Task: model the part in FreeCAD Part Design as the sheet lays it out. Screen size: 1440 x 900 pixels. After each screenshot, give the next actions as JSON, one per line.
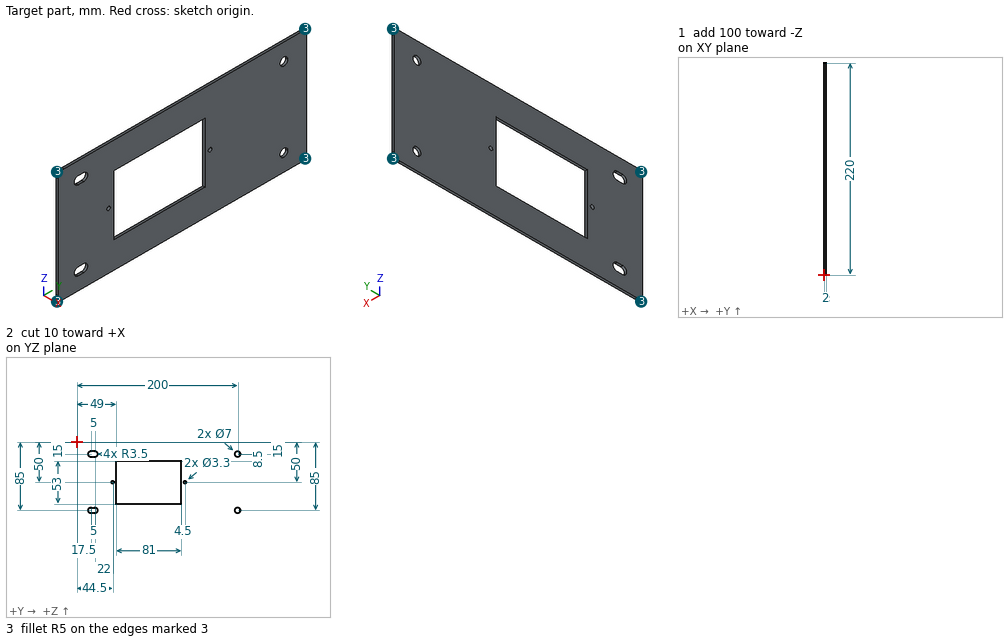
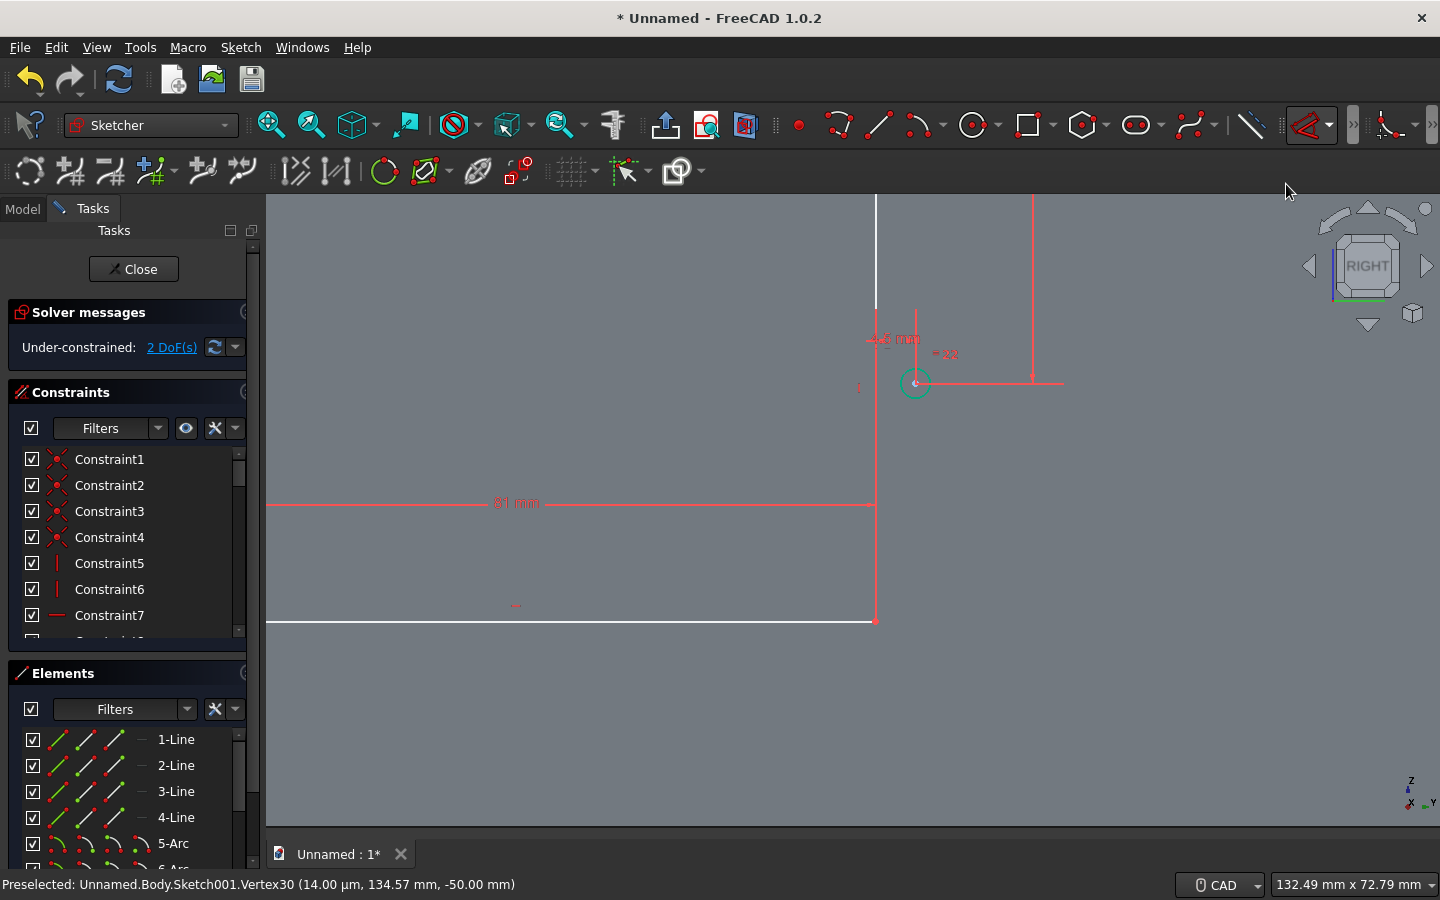
{"action": "scroll", "coordinate": [877, 624], "scroll_direction": "down", "scroll_amount": 5}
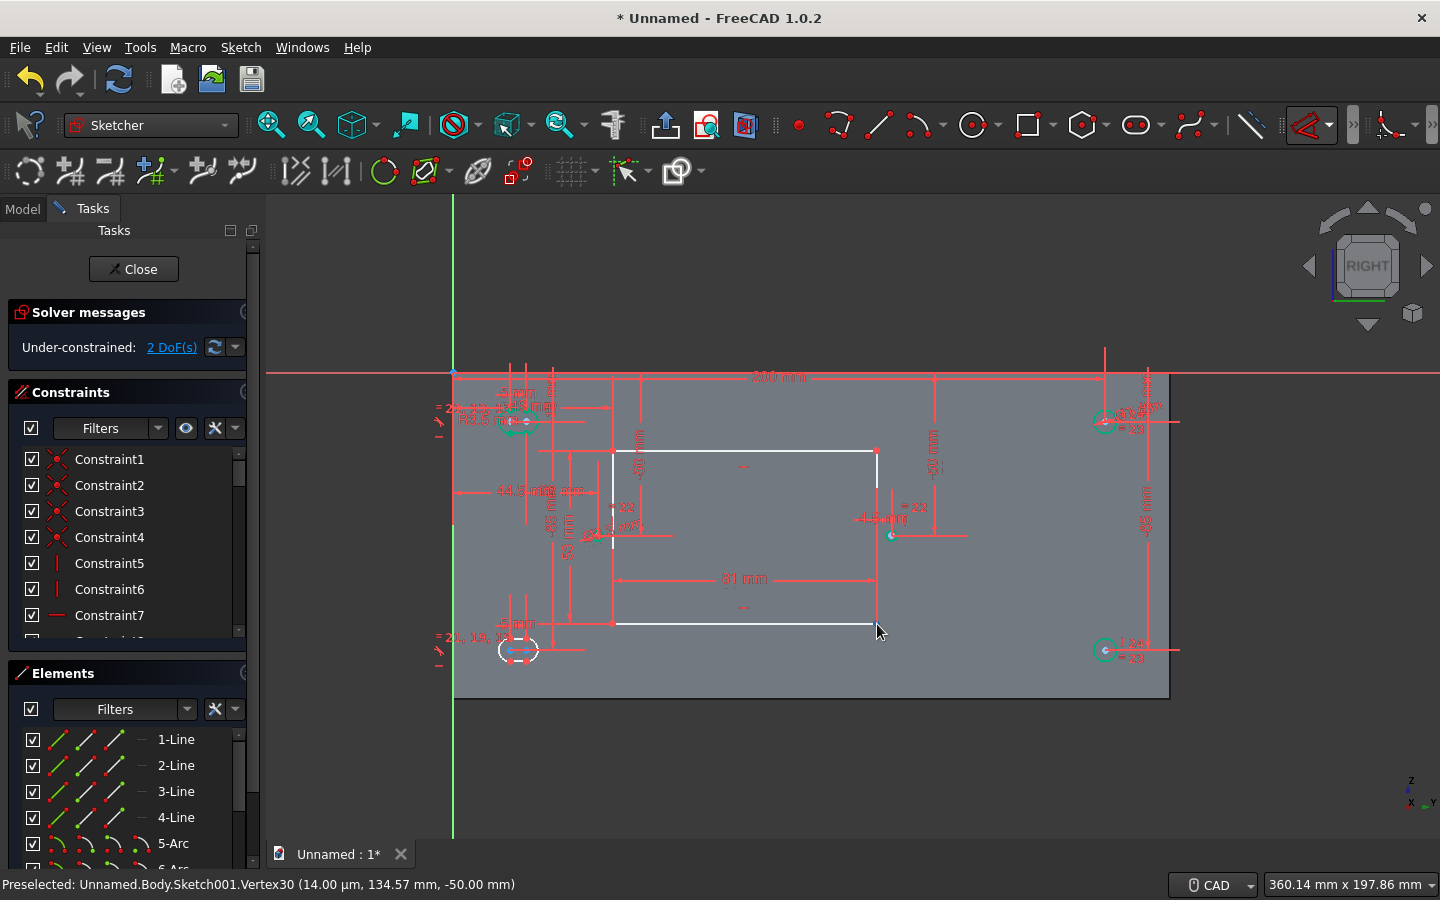
{"action": "scroll", "coordinate": [877, 451], "scroll_direction": "up", "scroll_amount": 2}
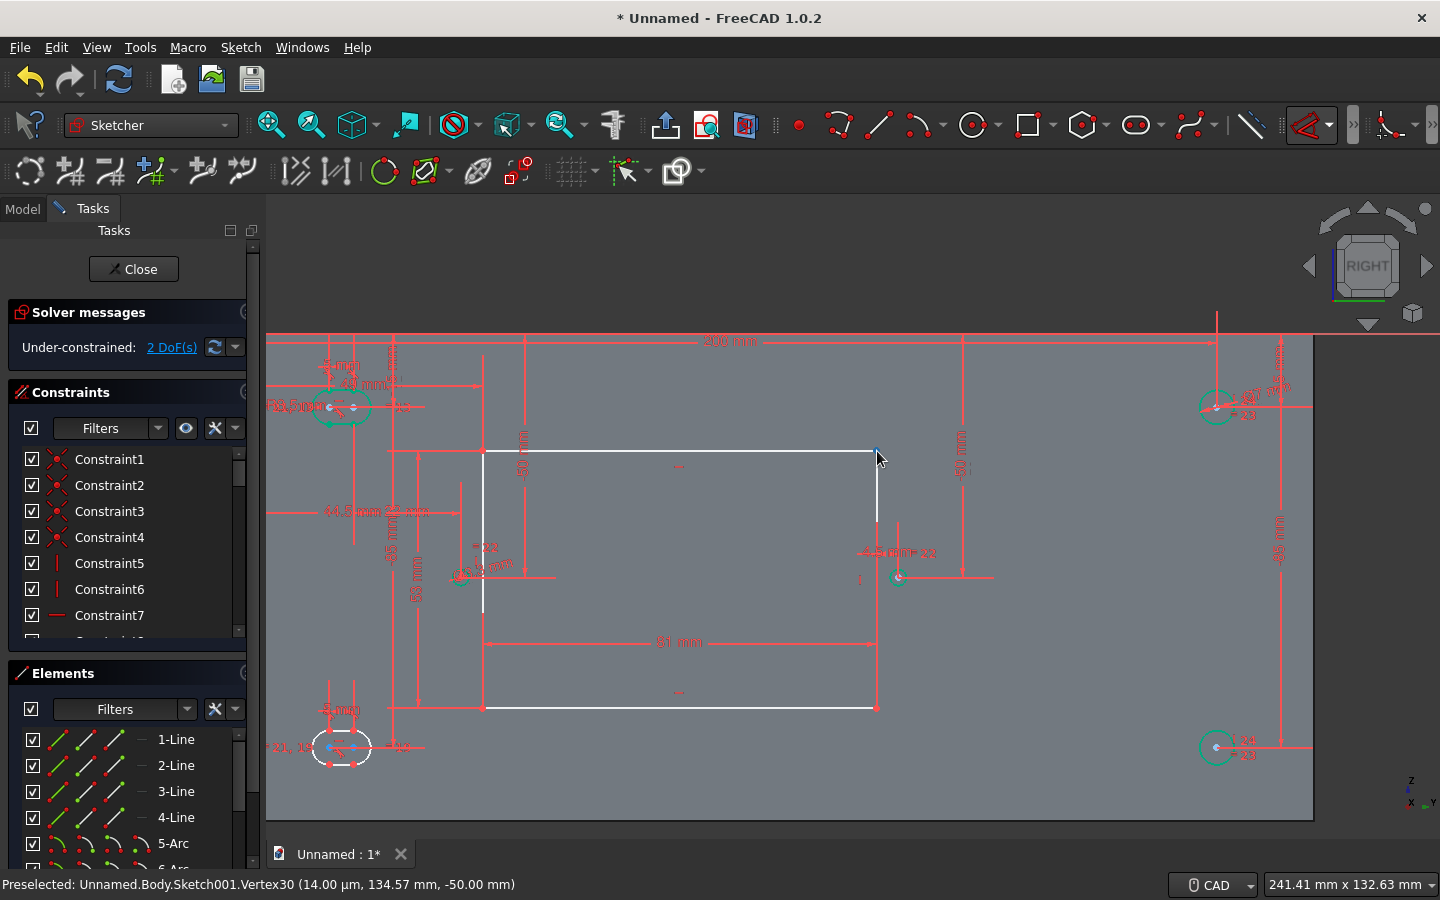
{"action": "left_click", "coordinate": [877, 451]}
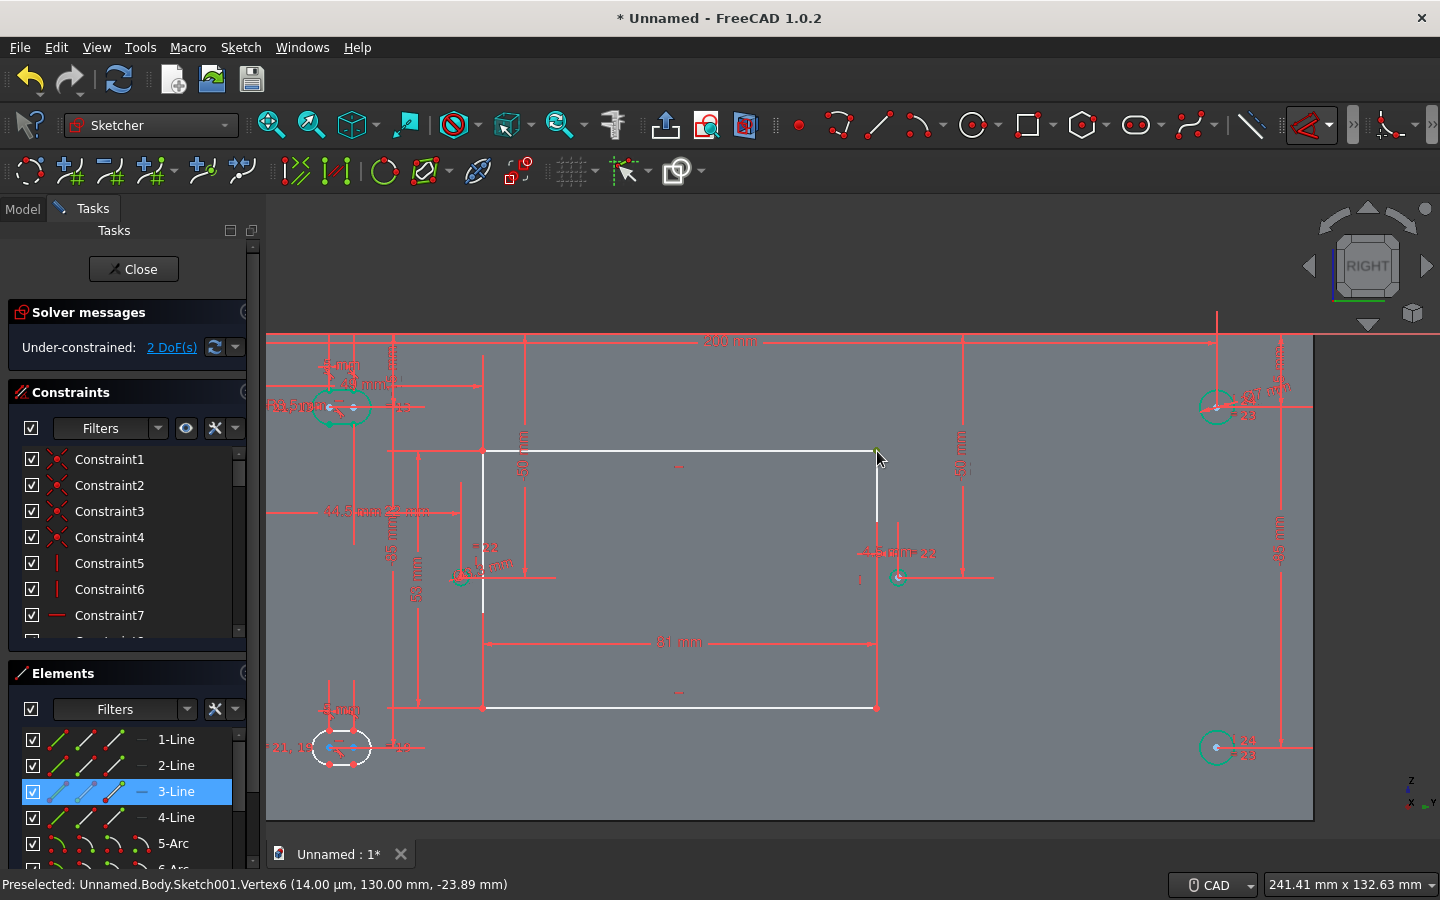
{"action": "left_click", "coordinate": [1217, 407]}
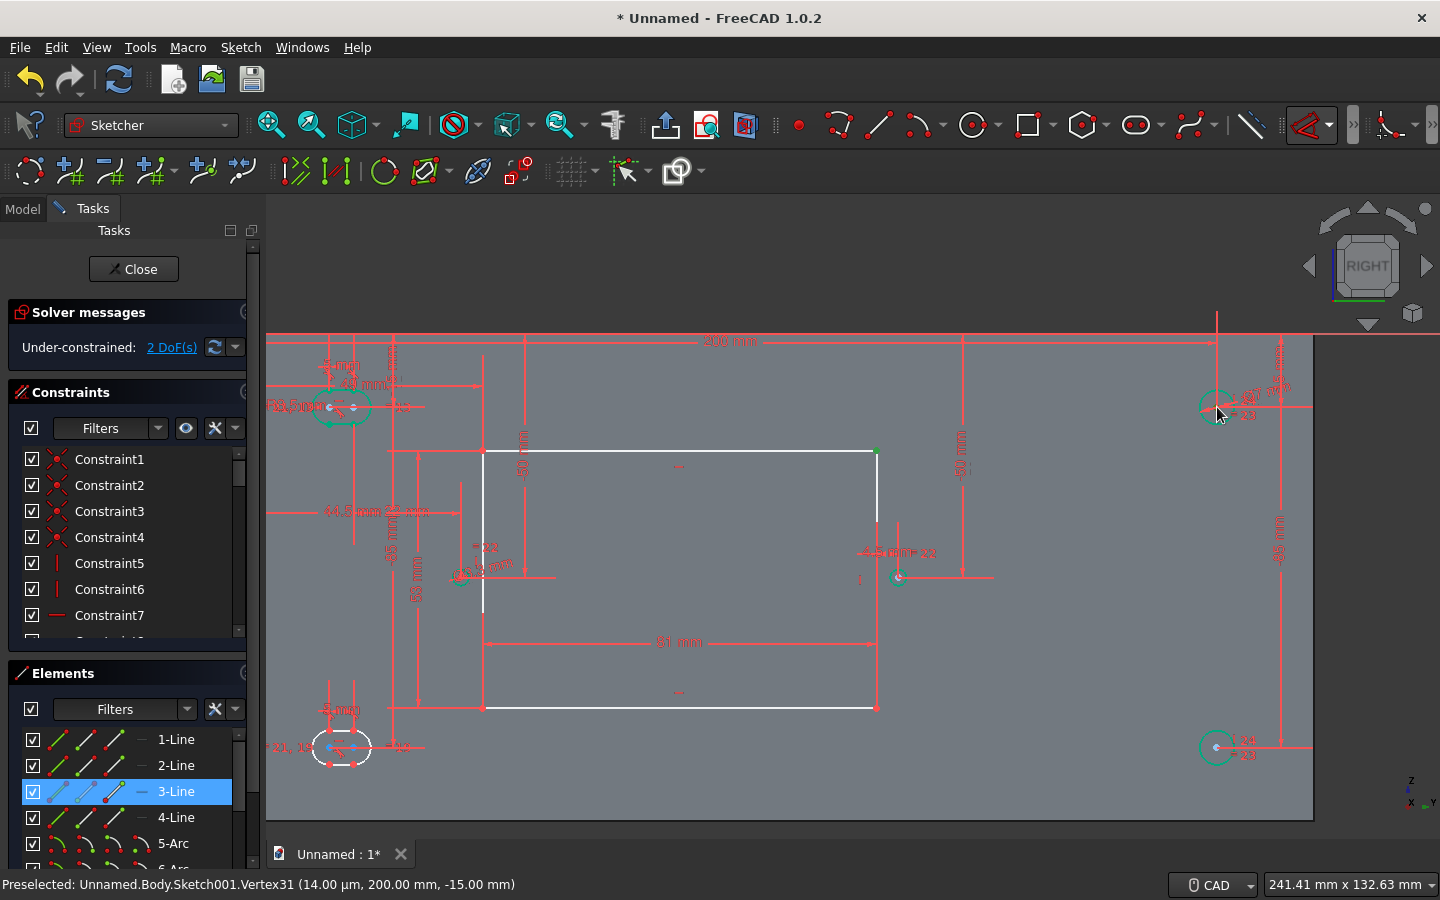
{"action": "key", "text": "i"}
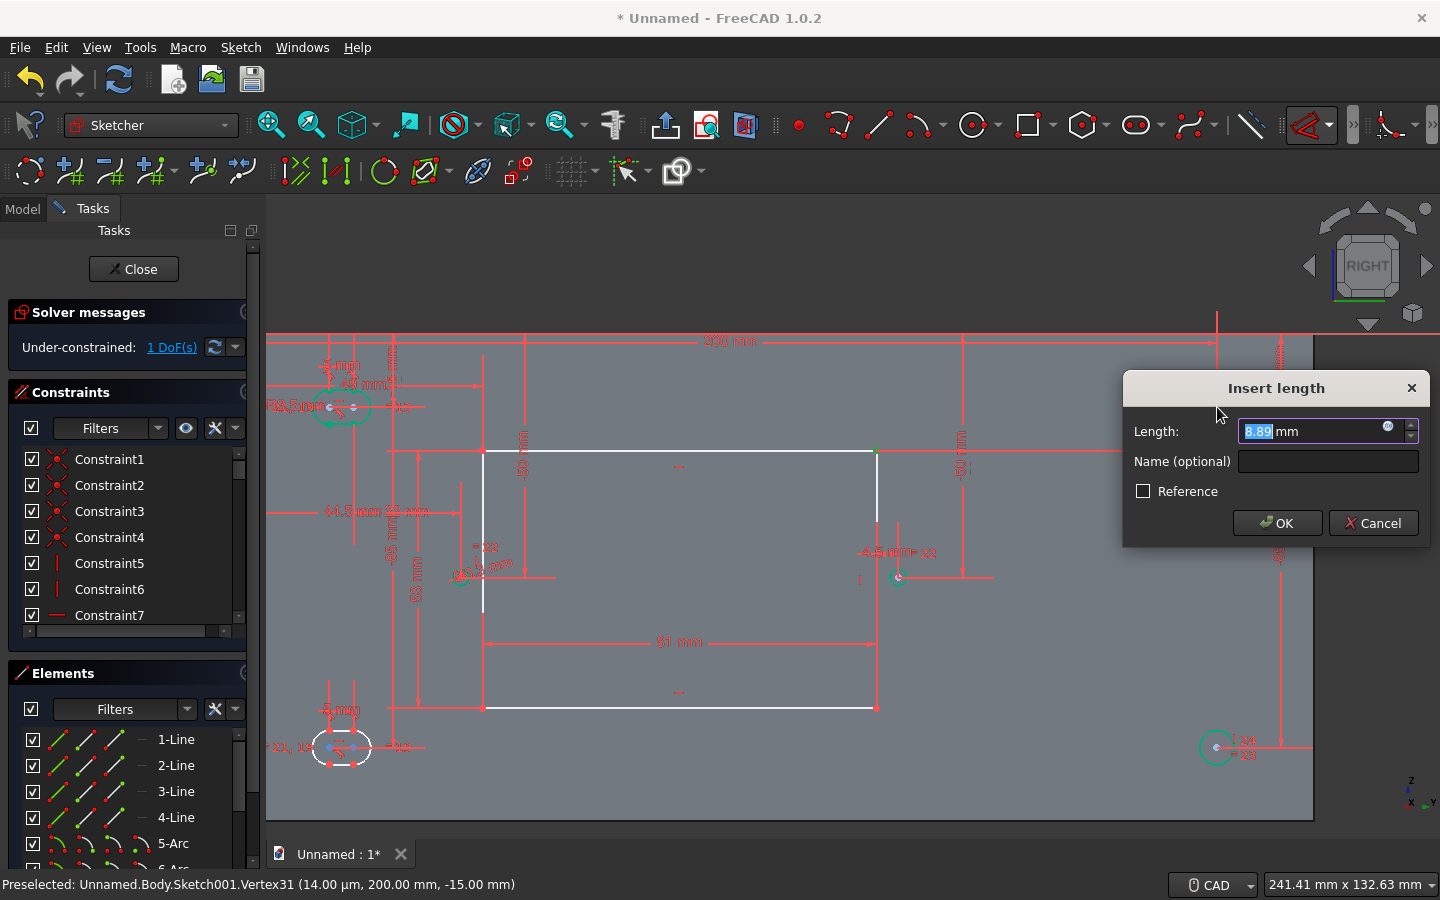
{"action": "type", "text": "8.5"}
{"action": "key", "text": "Return"}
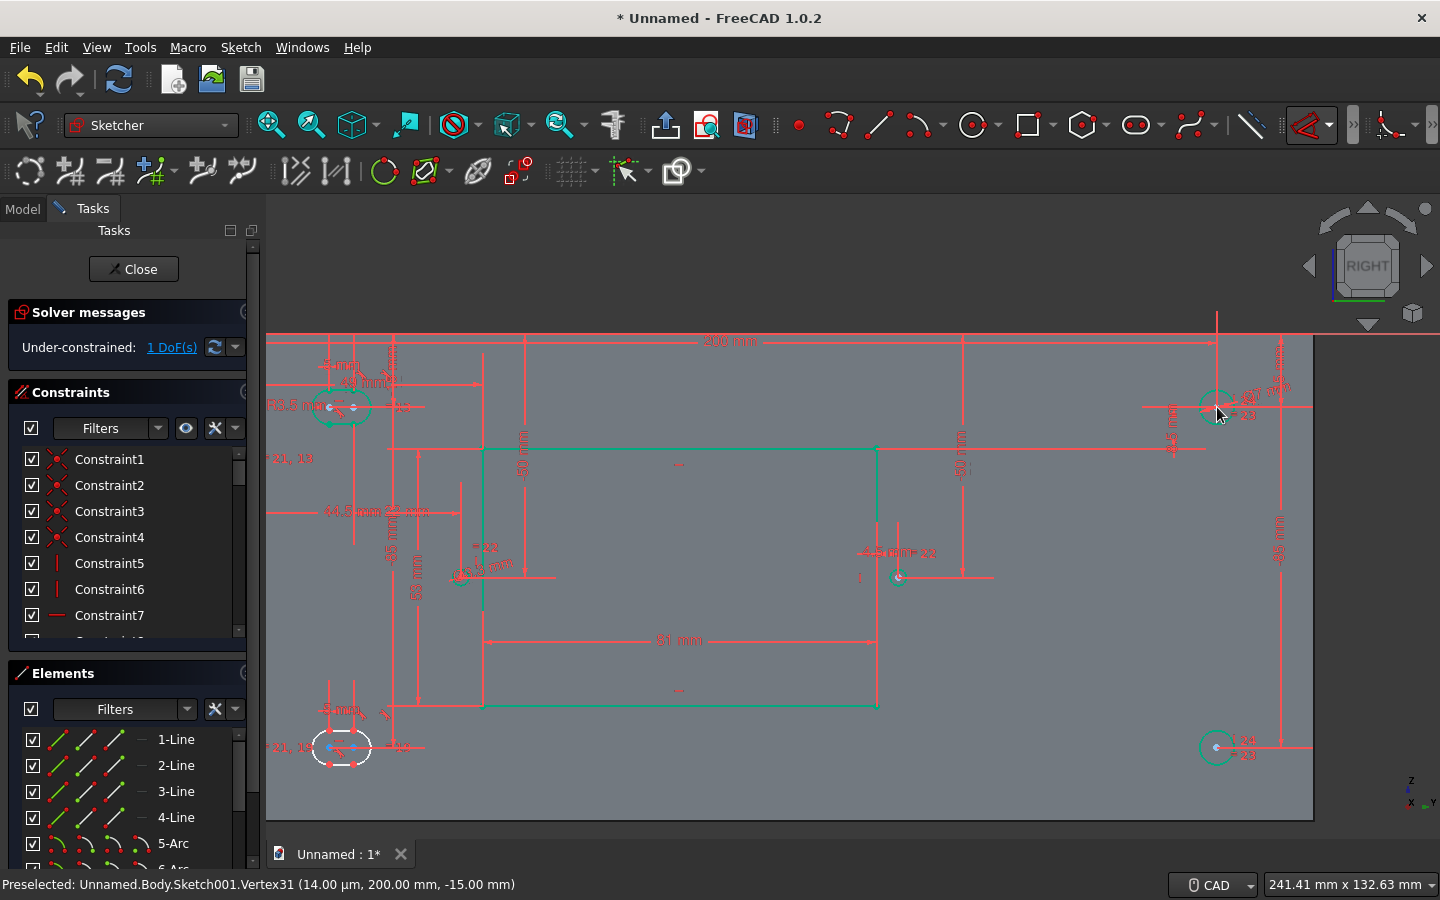
{"action": "left_click", "coordinate": [329, 731]}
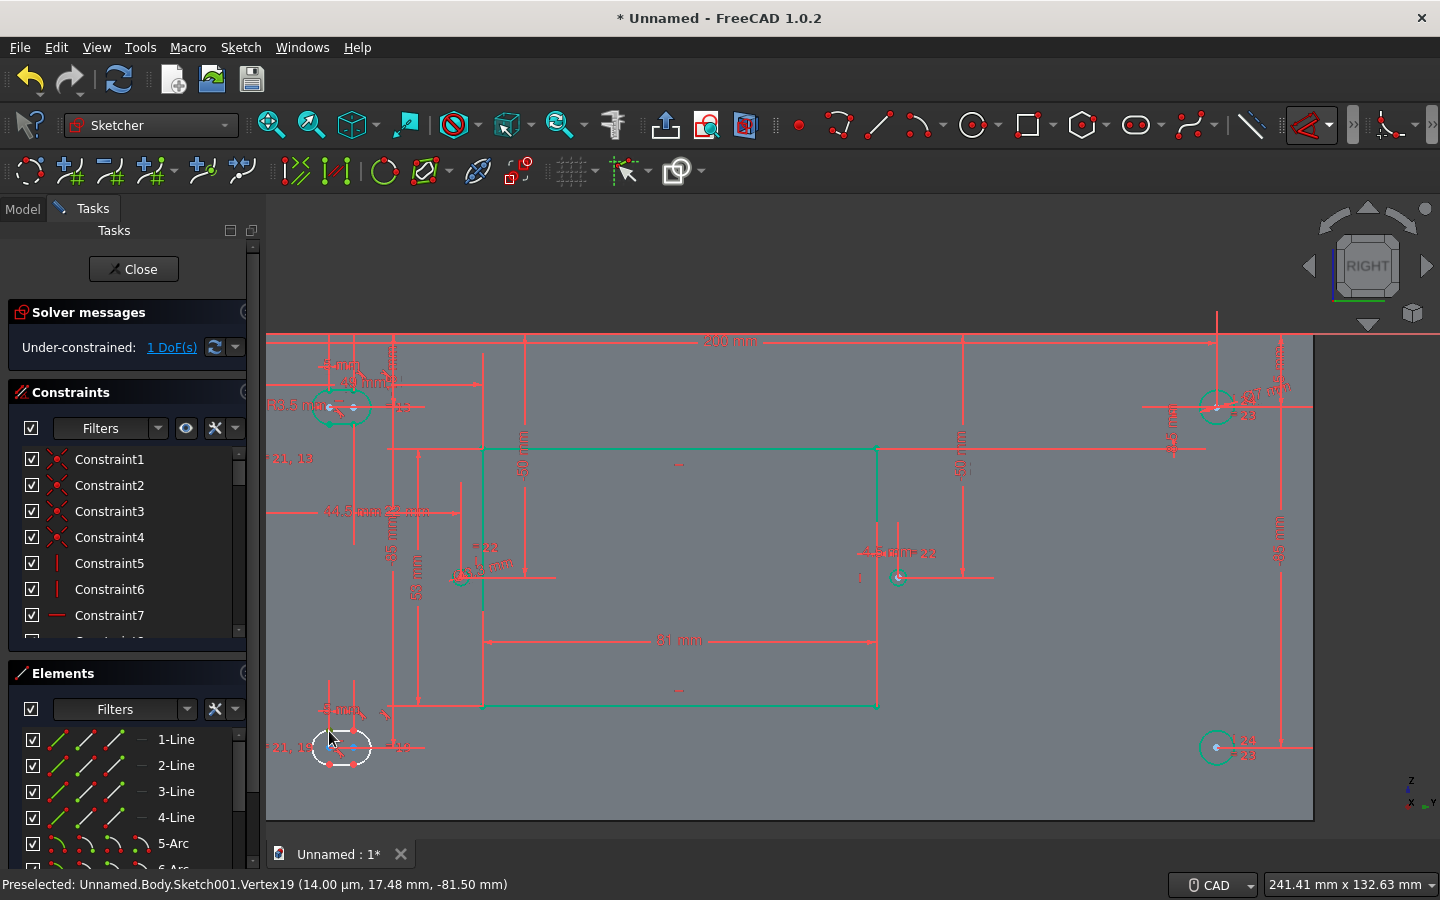
{"action": "left_click", "coordinate": [1332, 126]}